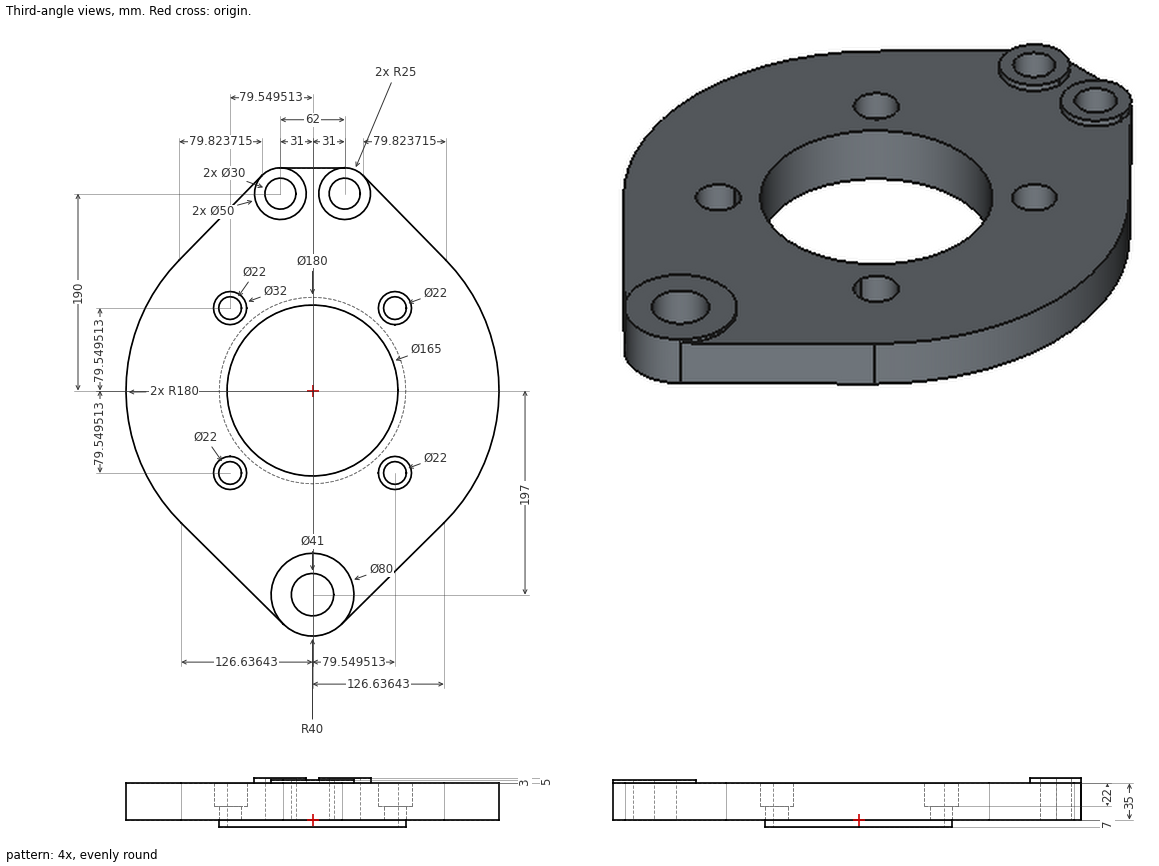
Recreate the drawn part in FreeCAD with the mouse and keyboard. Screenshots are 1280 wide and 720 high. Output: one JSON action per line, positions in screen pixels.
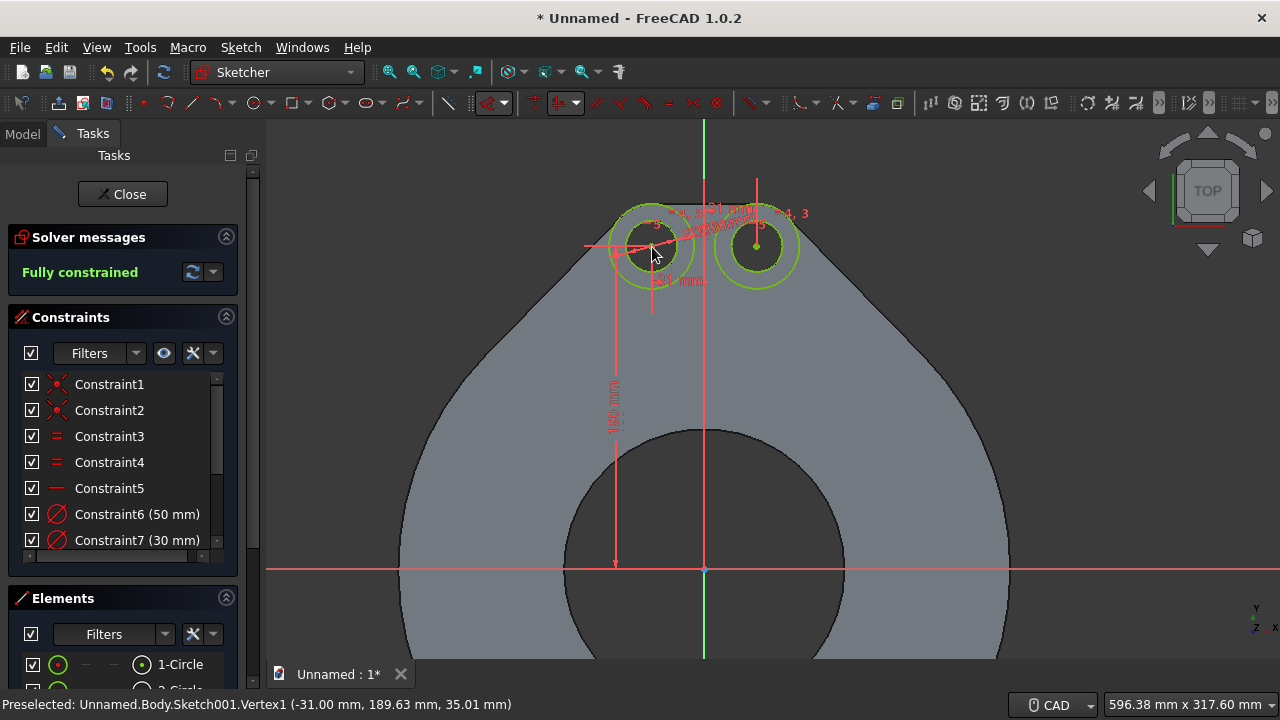
{"action": "left_click", "coordinate": [123, 194]}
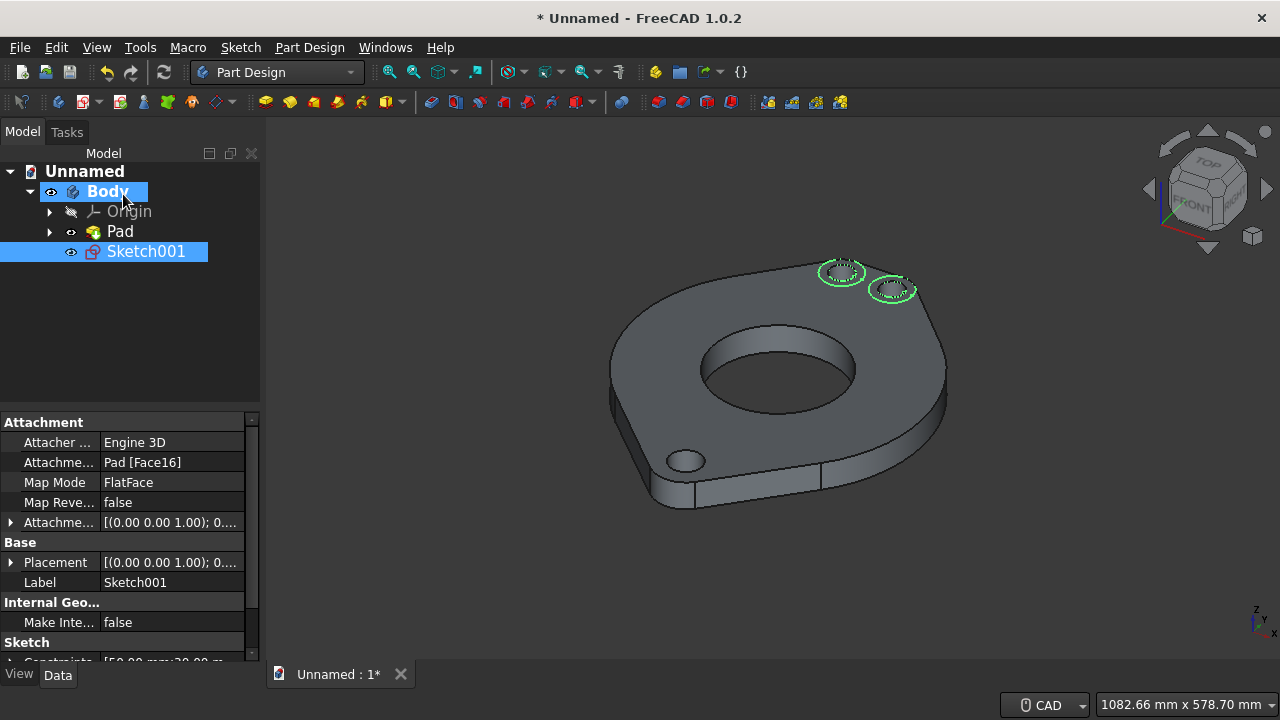
{"action": "left_click", "coordinate": [266, 102]}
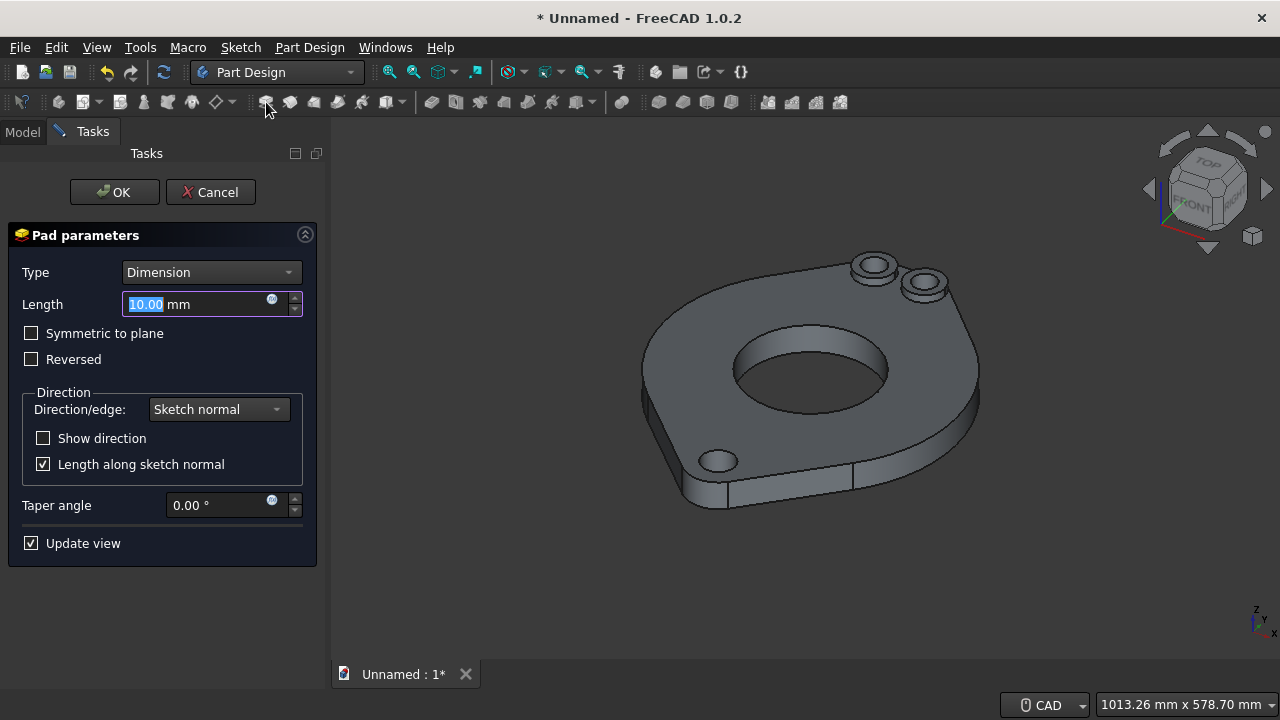
{"action": "type", "text": "5"}
{"action": "key", "text": "Tab"}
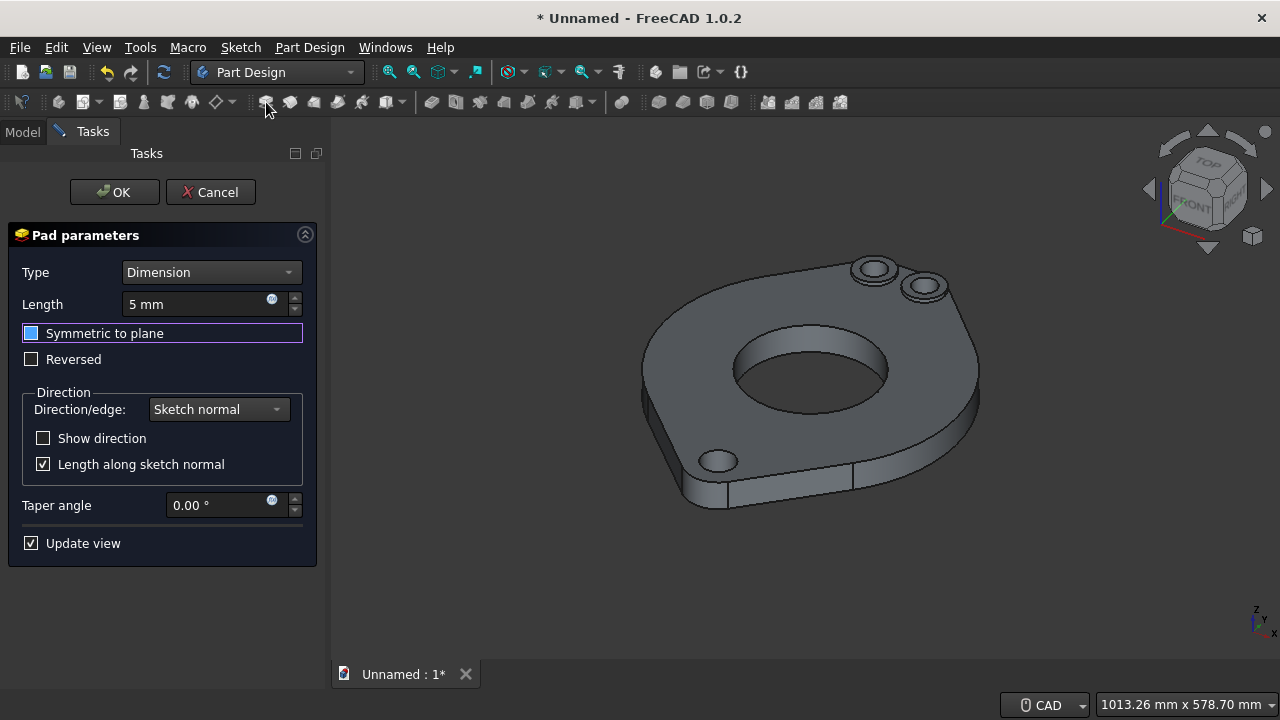
{"action": "left_click", "coordinate": [115, 192]}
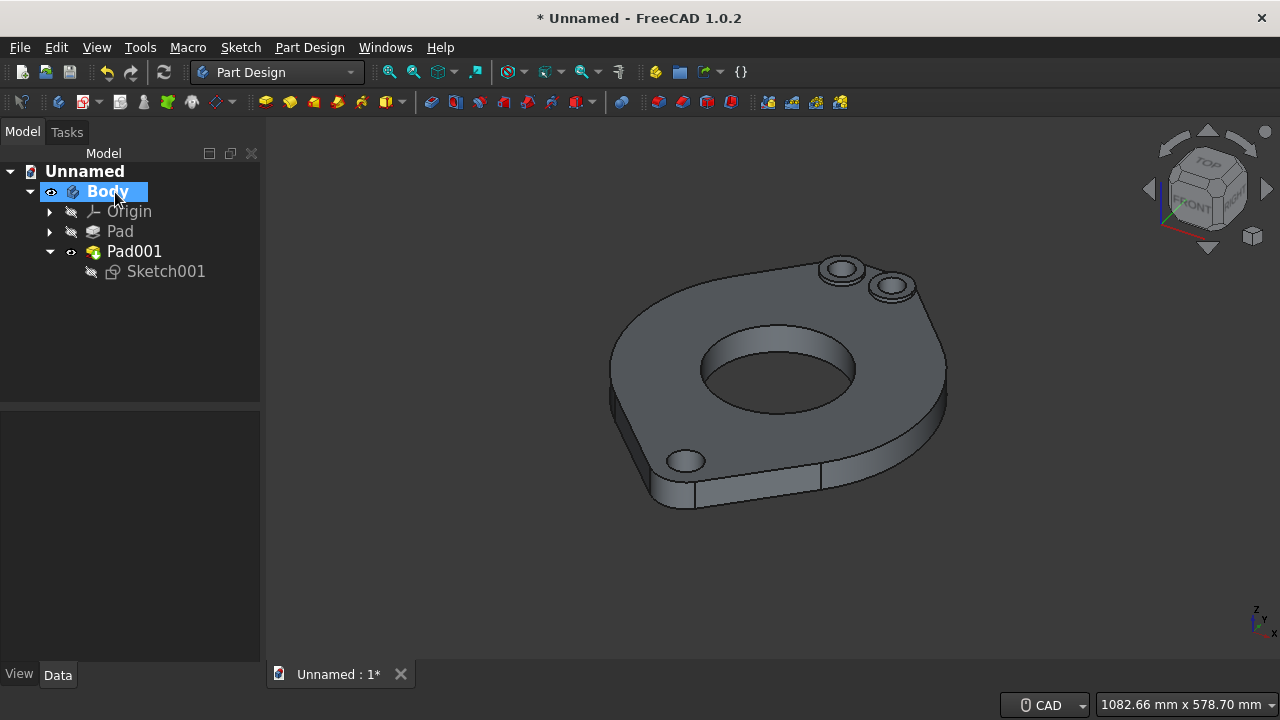
{"action": "left_click", "coordinate": [875, 327]}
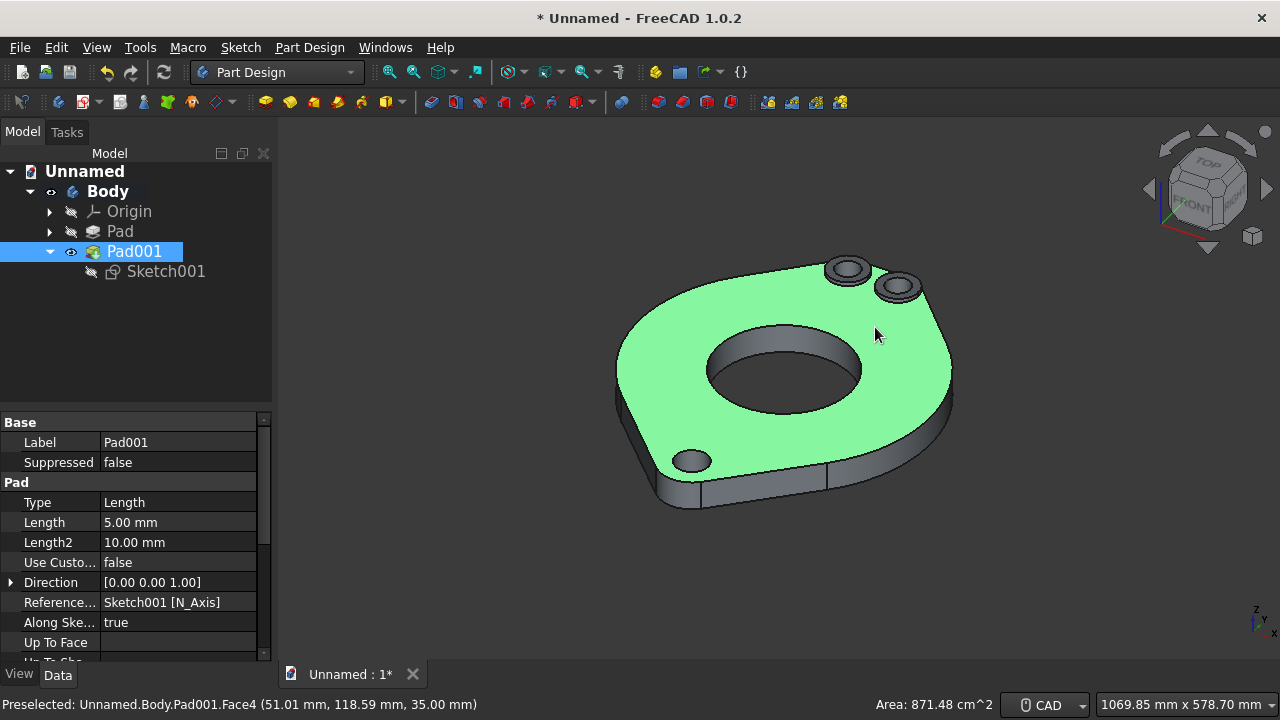
{"action": "left_click", "coordinate": [84, 102]}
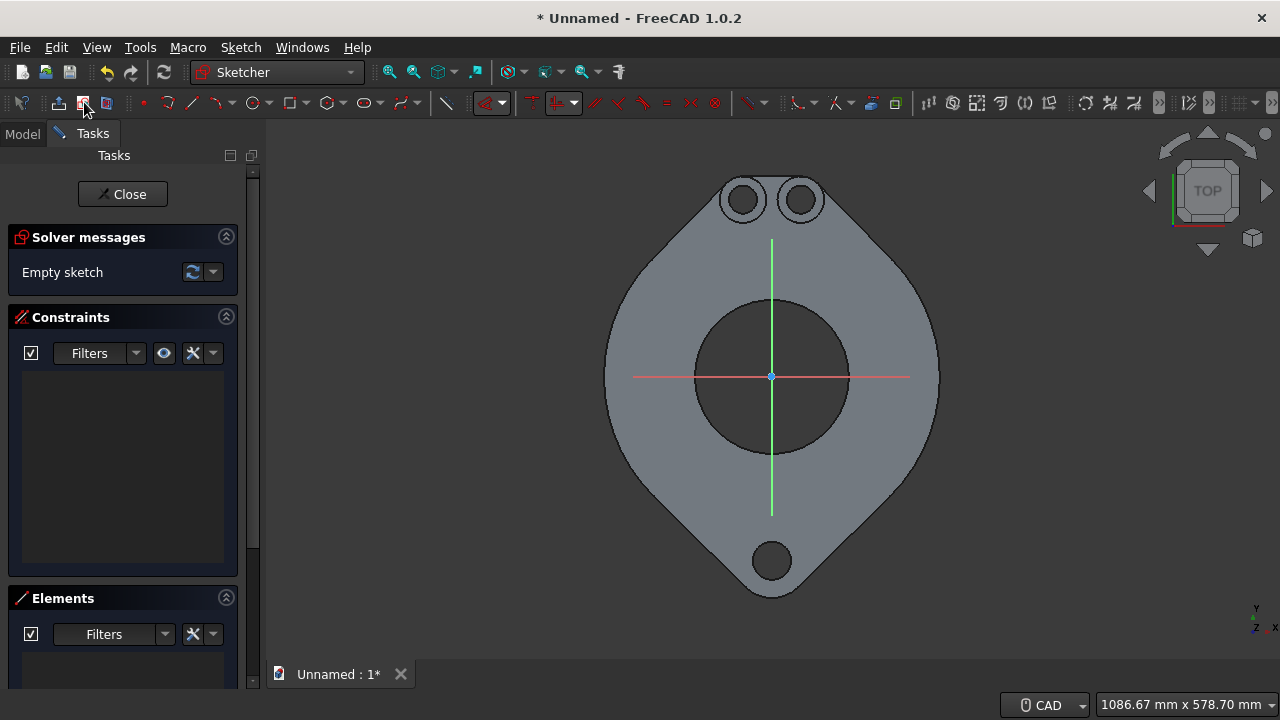
{"action": "key", "text": "q s"}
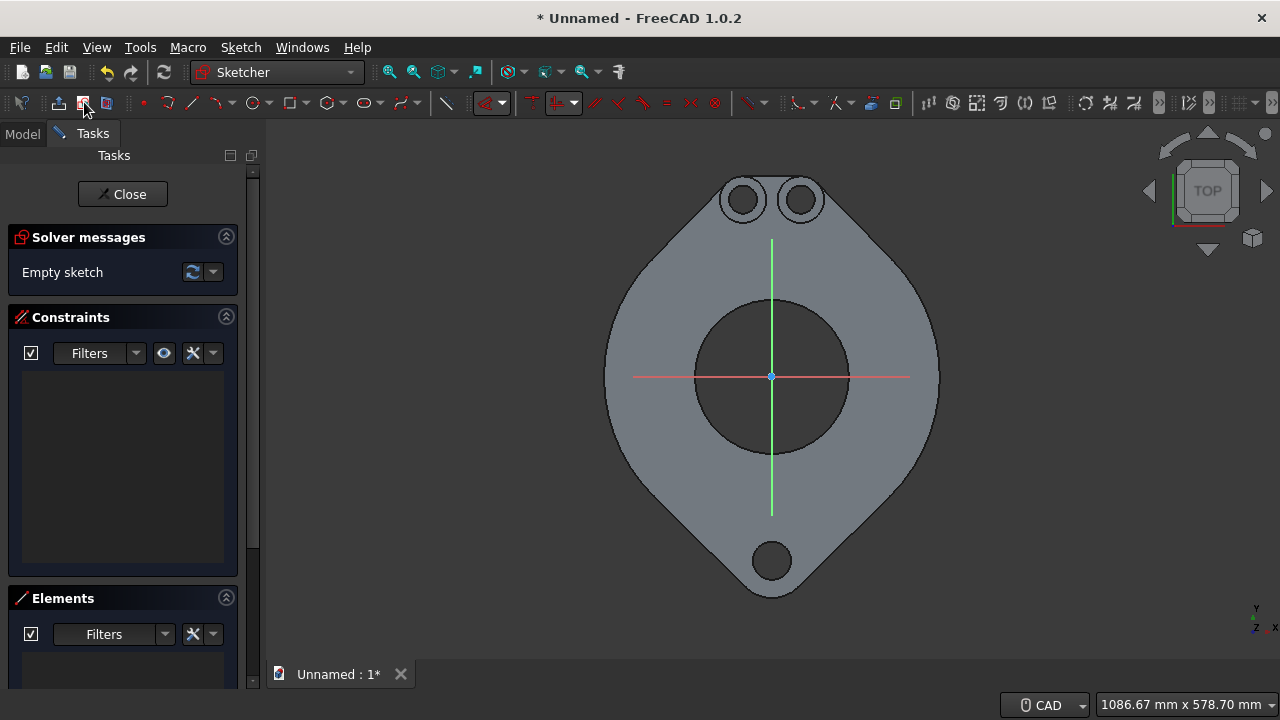
{"action": "scroll", "coordinate": [697, 297], "scroll_direction": "up", "scroll_amount": 14}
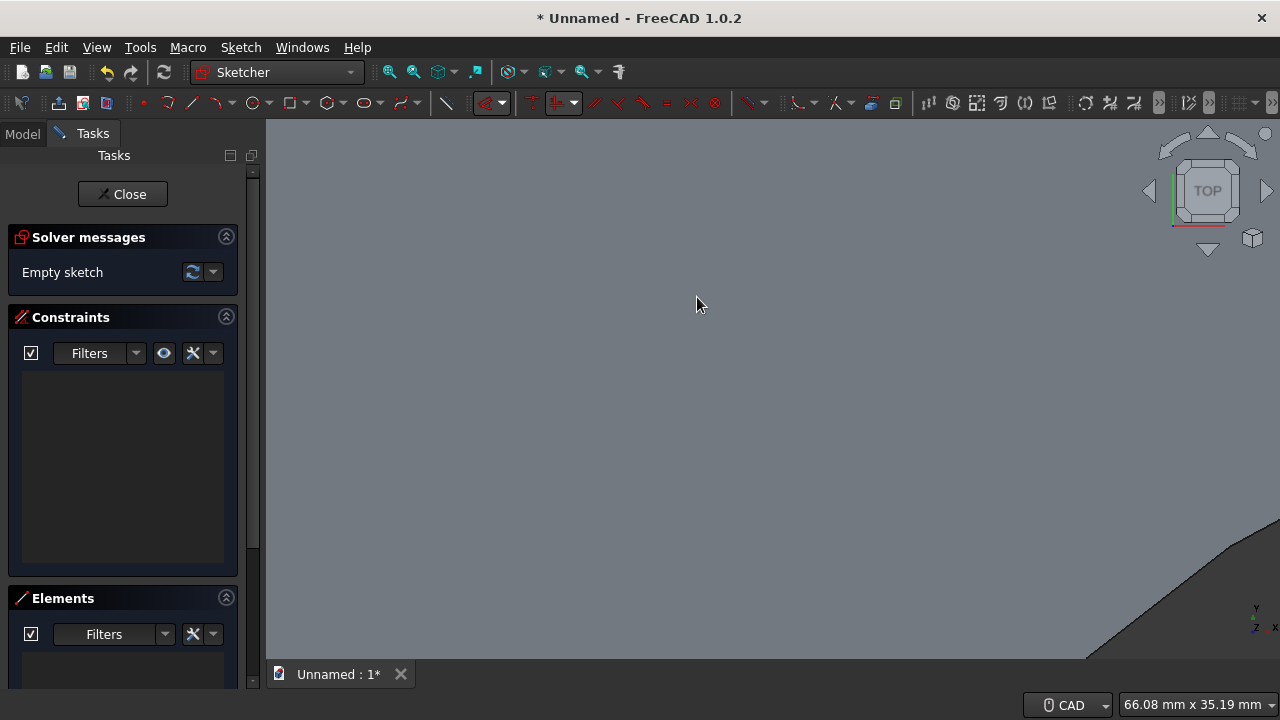
{"action": "key", "text": "g c"}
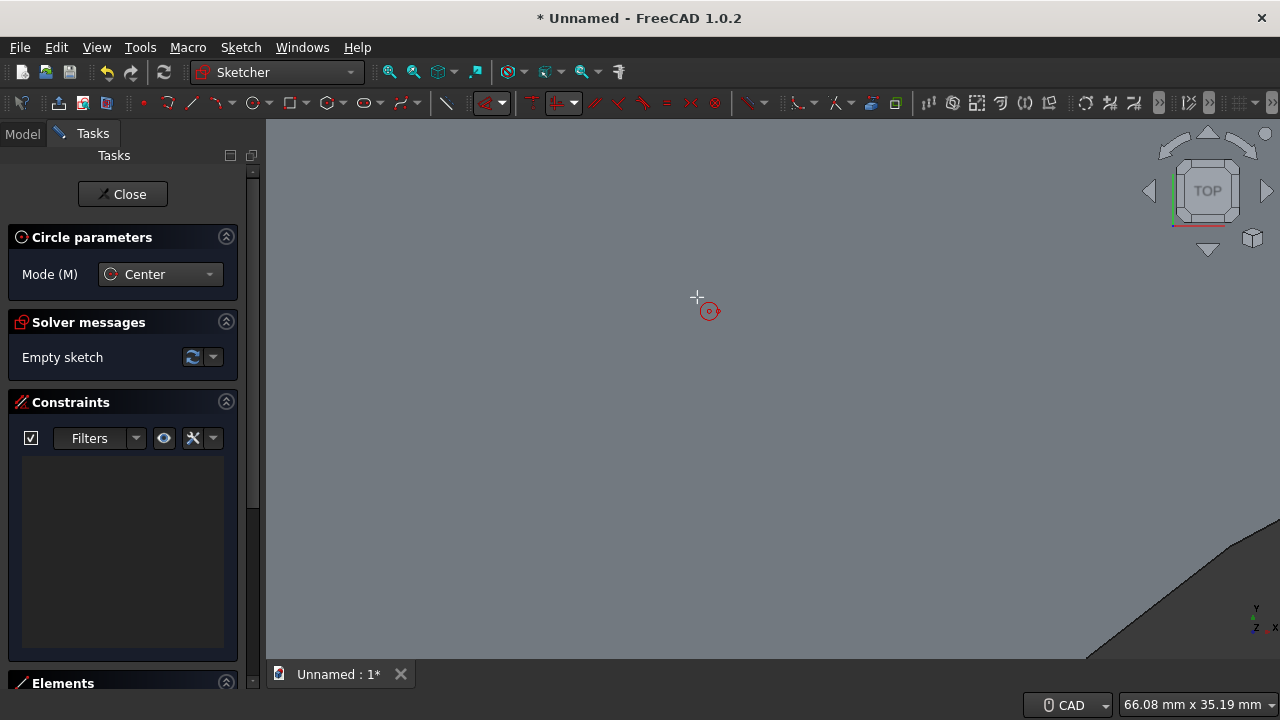
{"action": "left_click", "coordinate": [702, 386]}
{"action": "left_click", "coordinate": [821, 267]}
{"action": "key", "text": "Escape"}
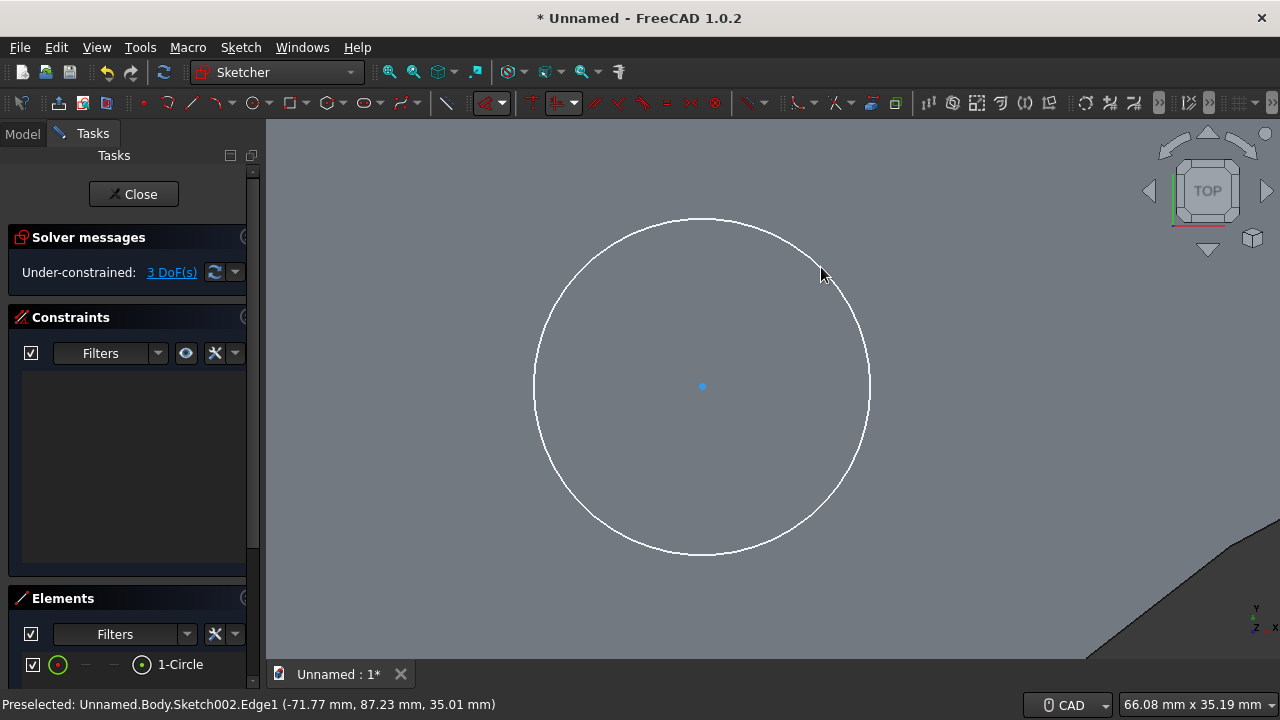
{"action": "left_click", "coordinate": [821, 268]}